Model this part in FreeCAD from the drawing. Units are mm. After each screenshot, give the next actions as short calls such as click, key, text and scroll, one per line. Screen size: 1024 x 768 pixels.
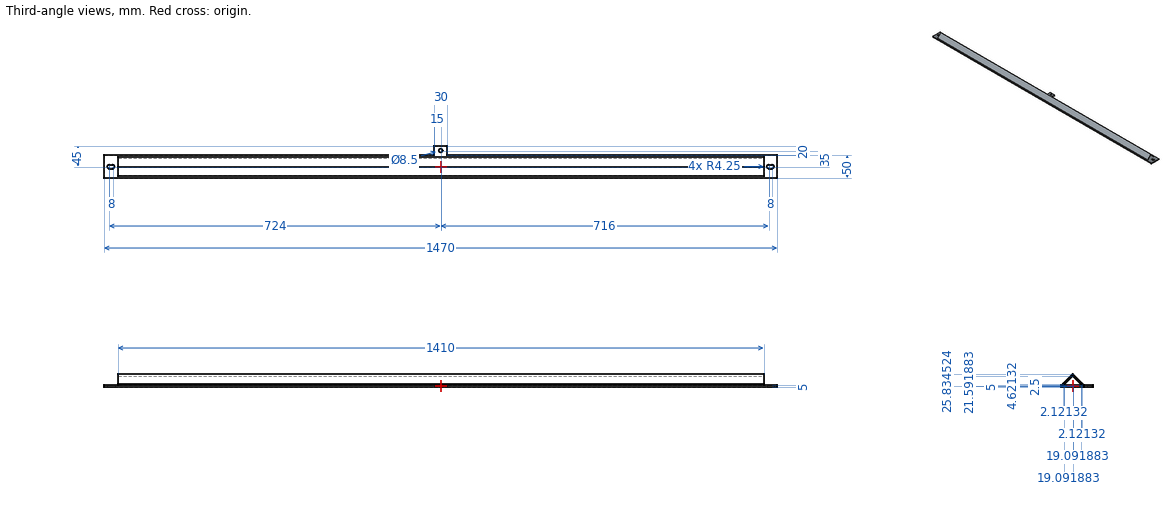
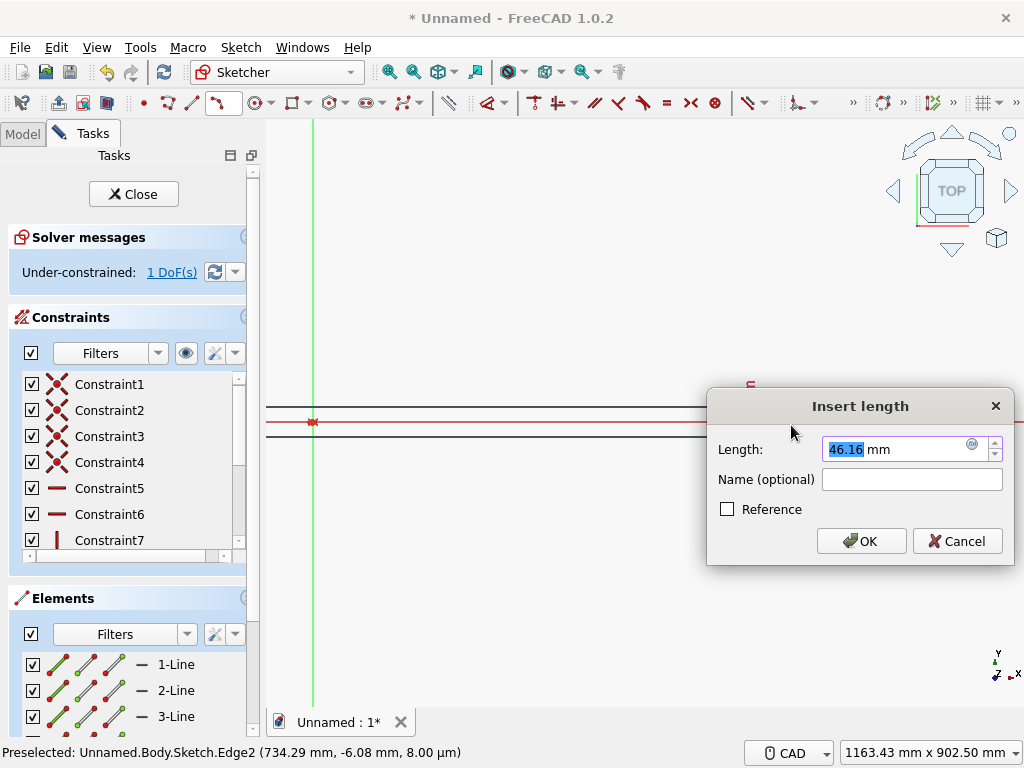
text(50)
key(Return)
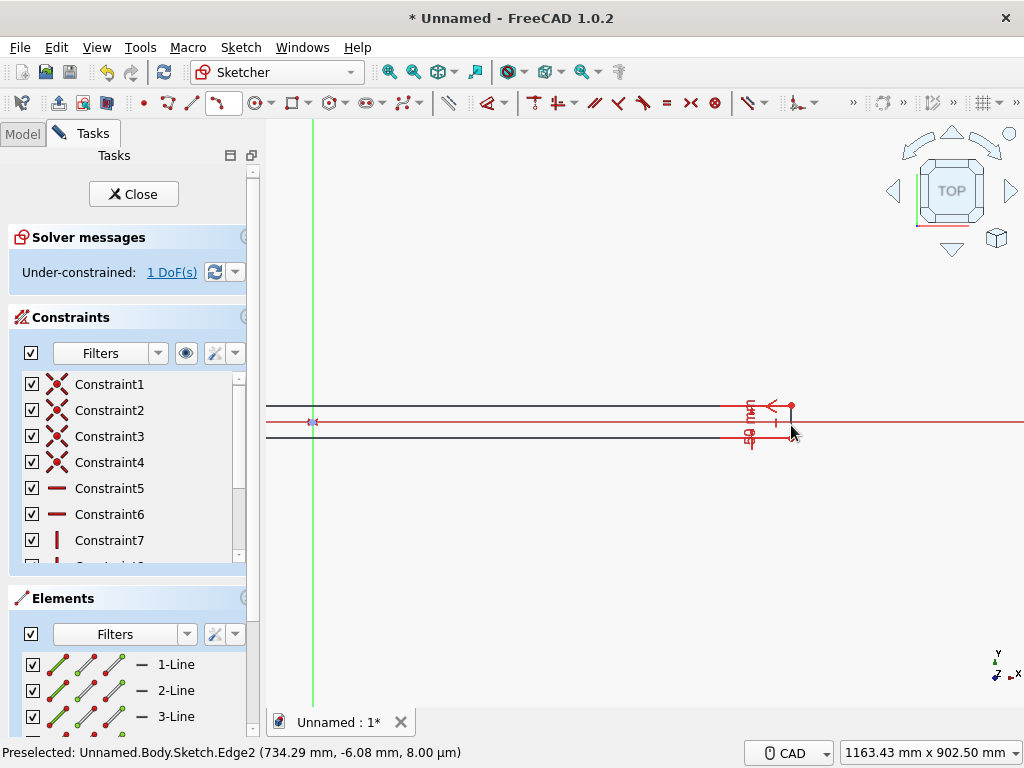
click(504, 438)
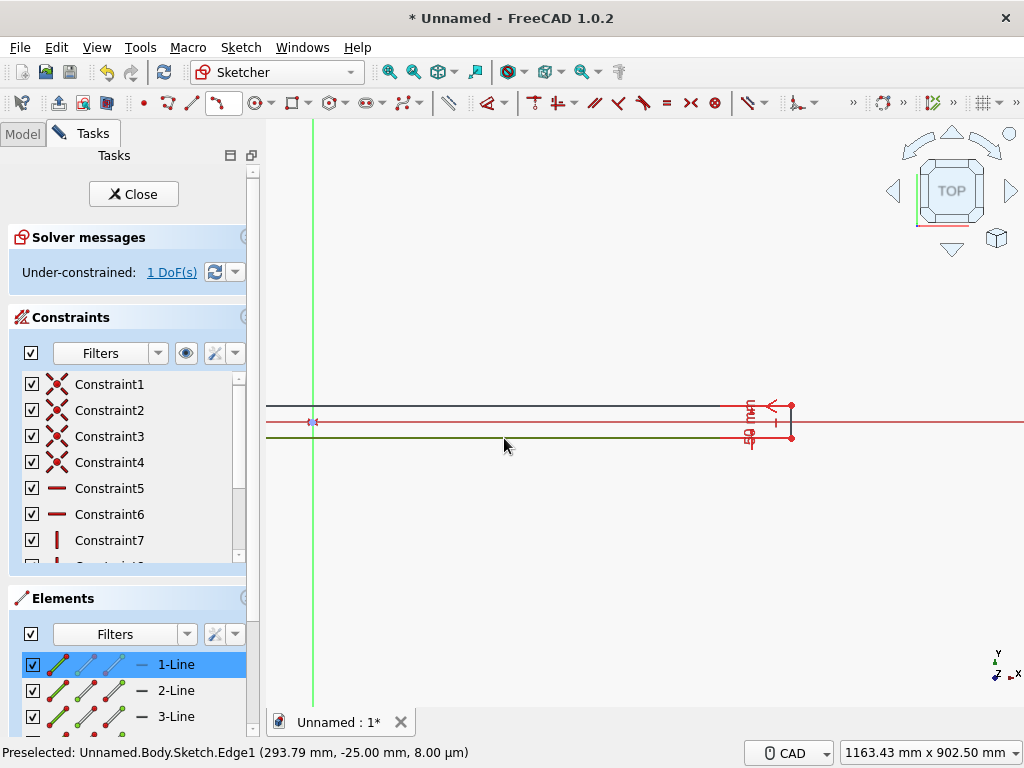
key(l)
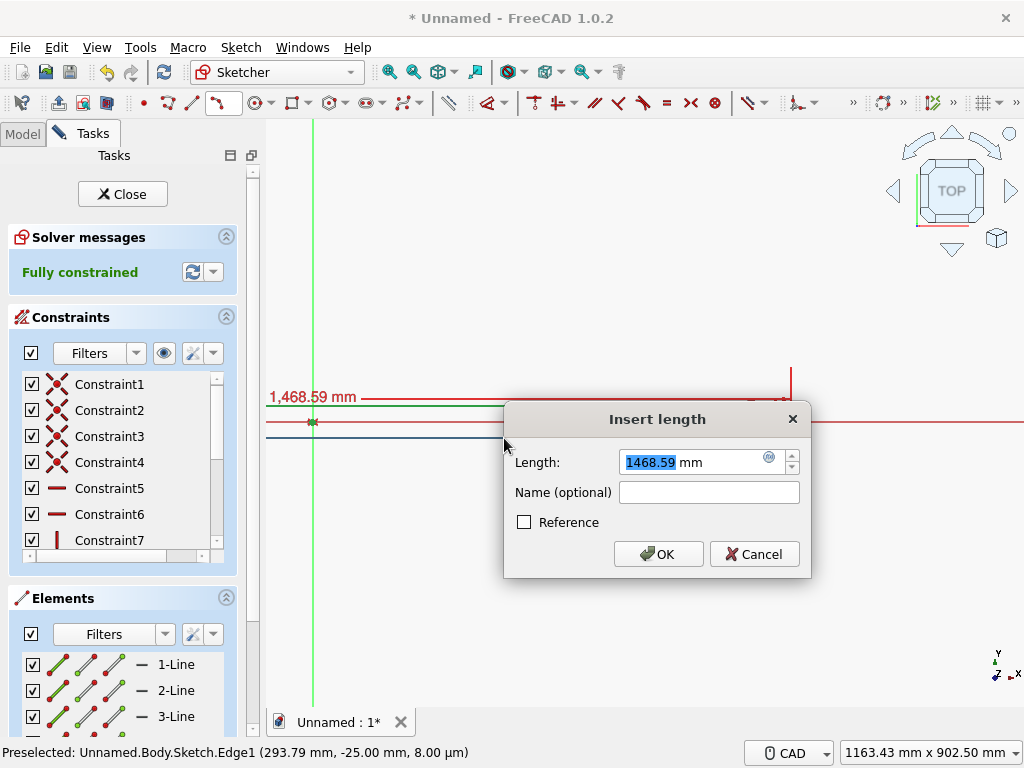
text(1470)
key(Return)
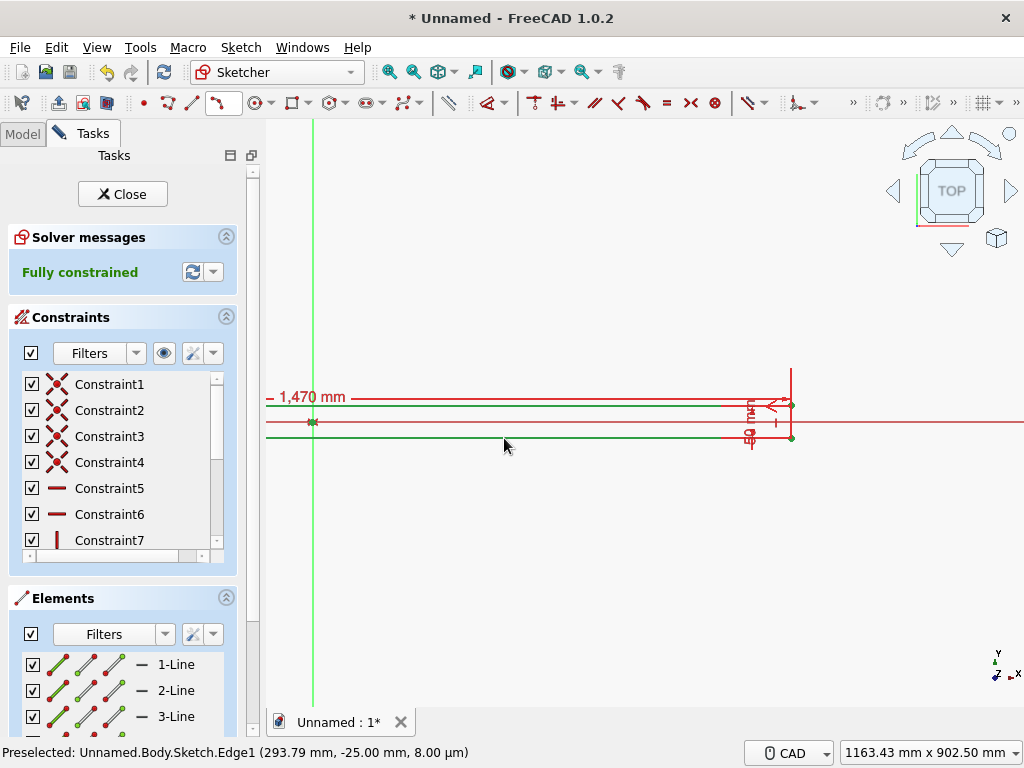
click(123, 194)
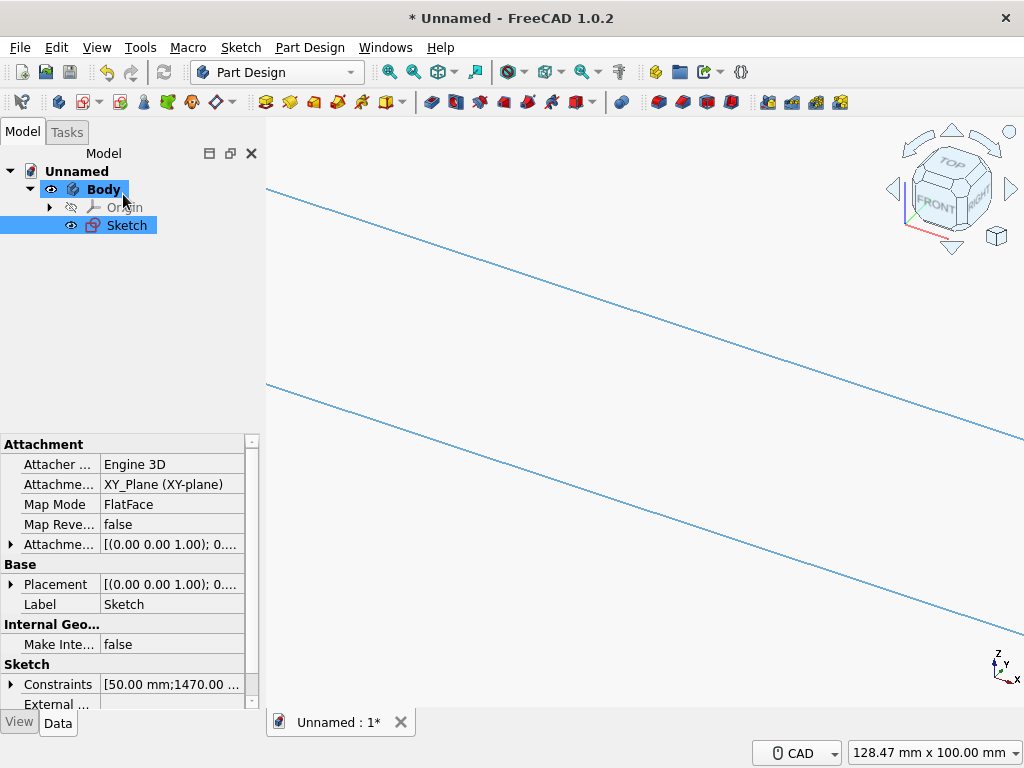
click(266, 102)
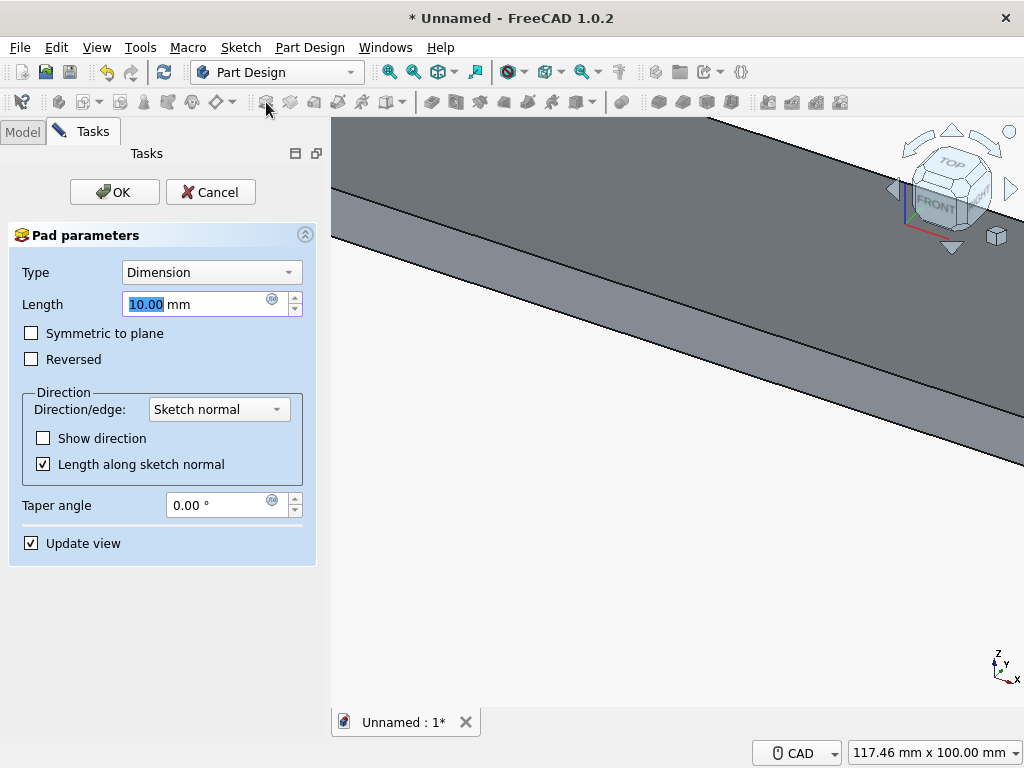
text(5)
key(Tab)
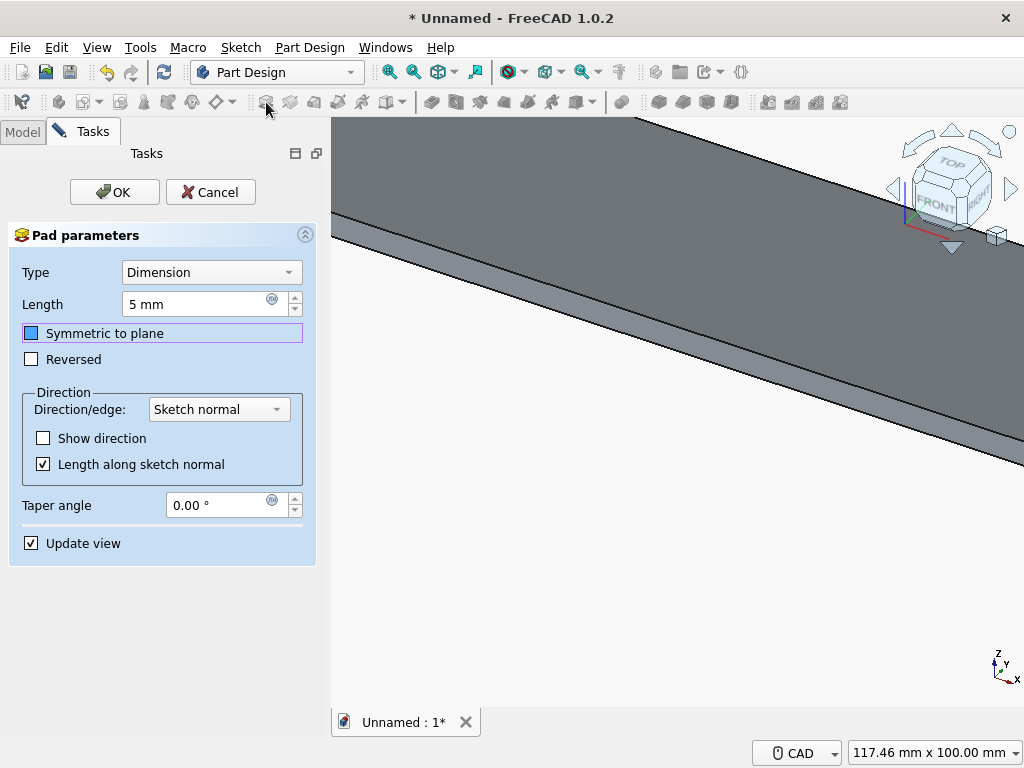
click(30, 333)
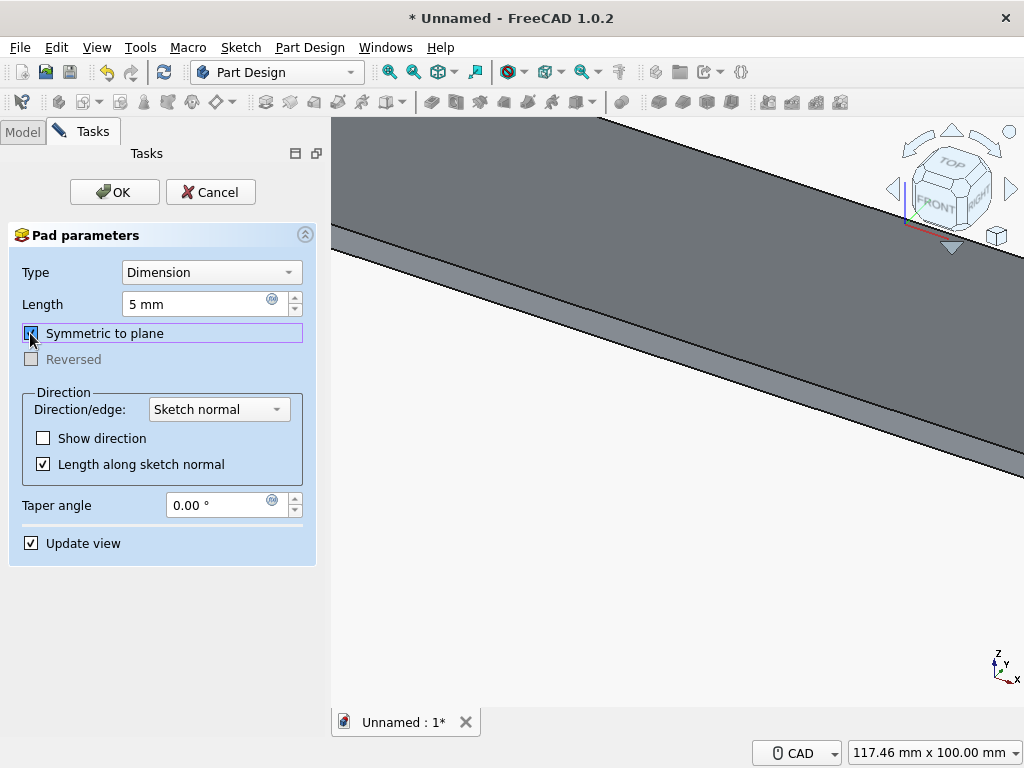
click(115, 192)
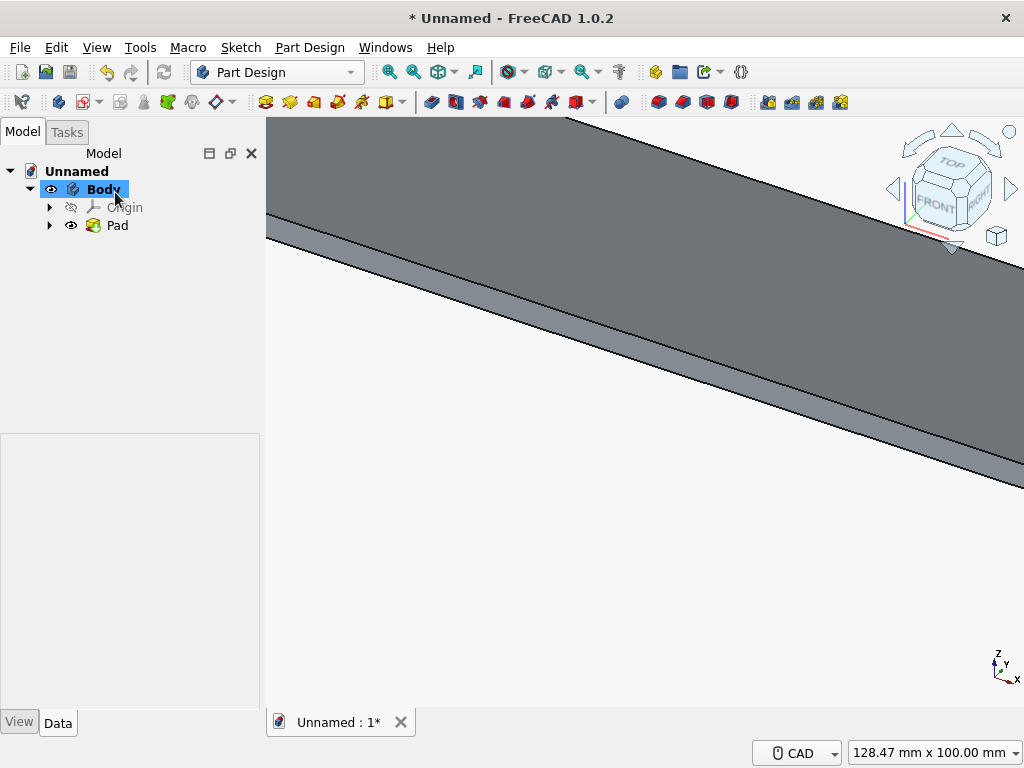
click(390, 72)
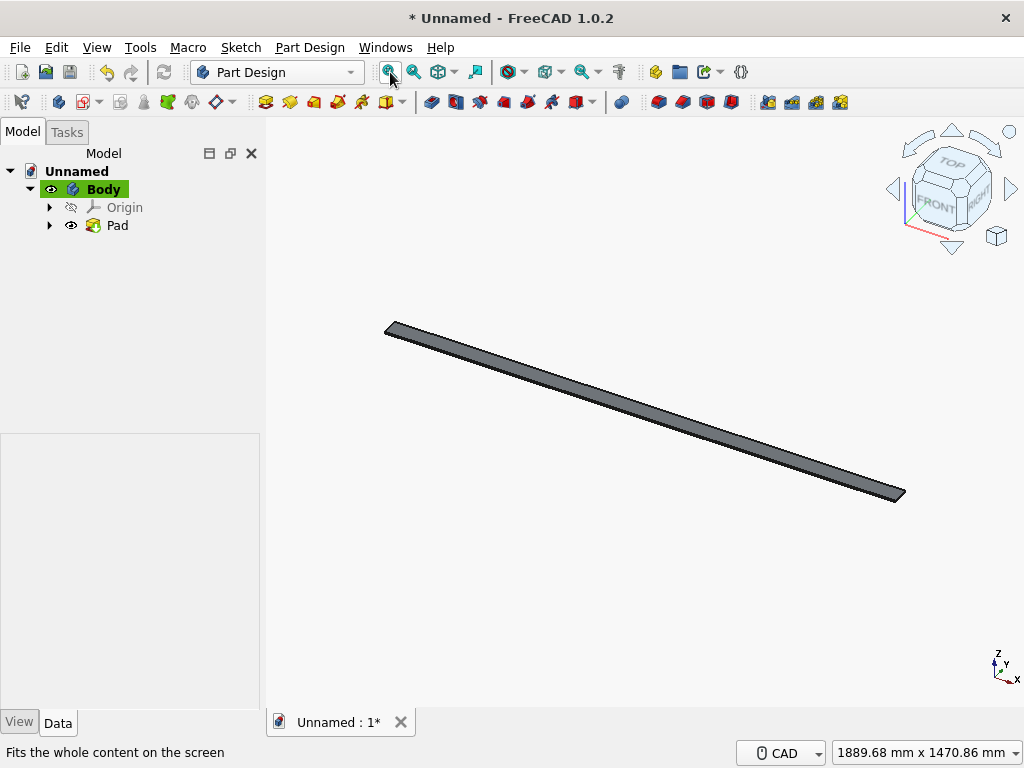
key(0)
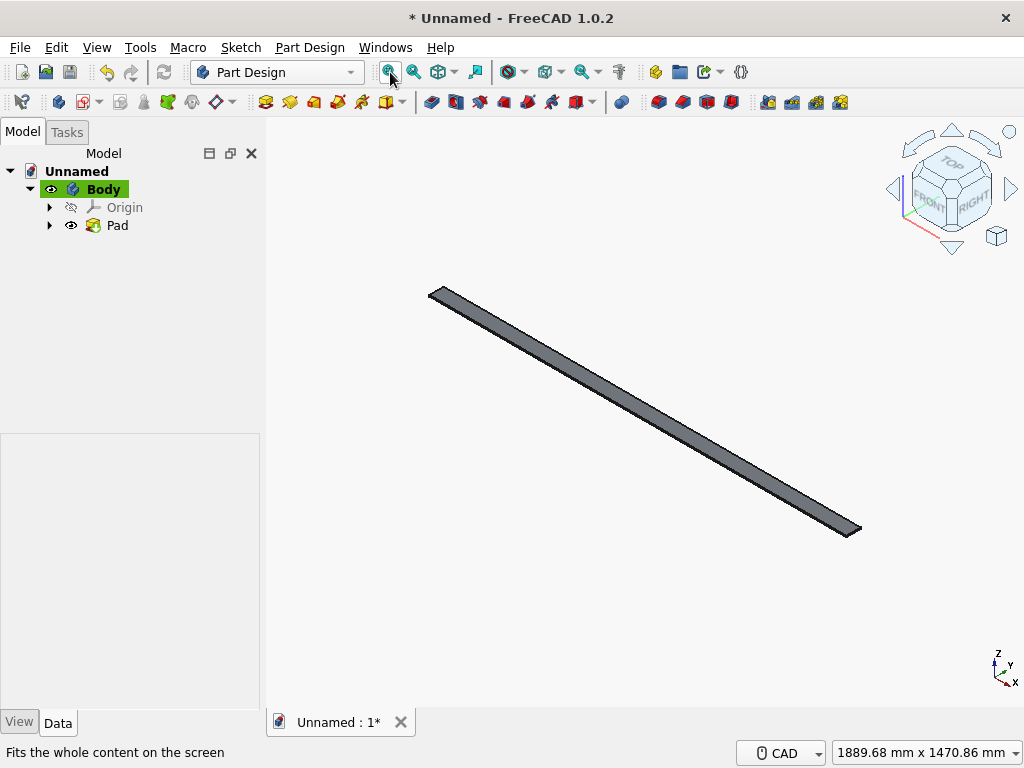
key(2)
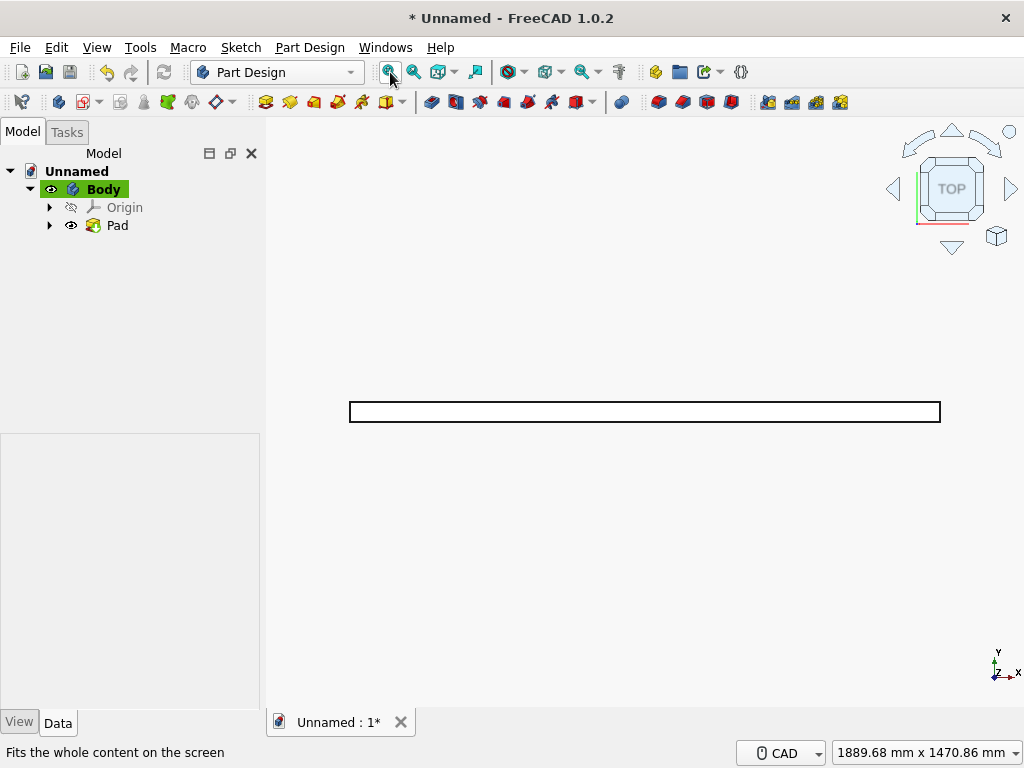
click(898, 411)